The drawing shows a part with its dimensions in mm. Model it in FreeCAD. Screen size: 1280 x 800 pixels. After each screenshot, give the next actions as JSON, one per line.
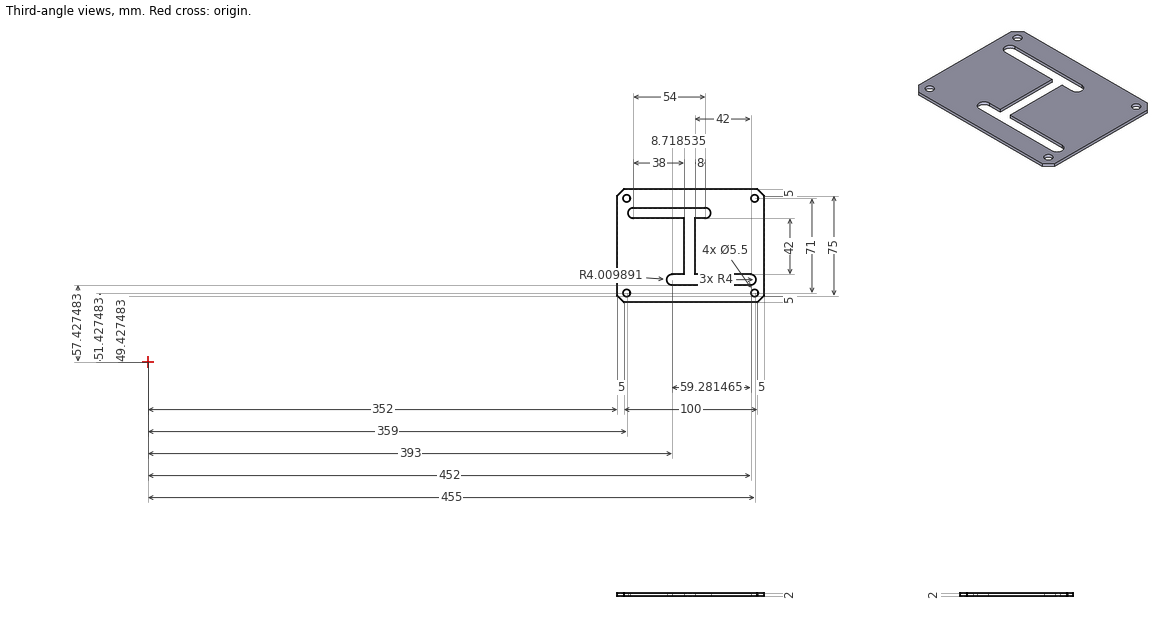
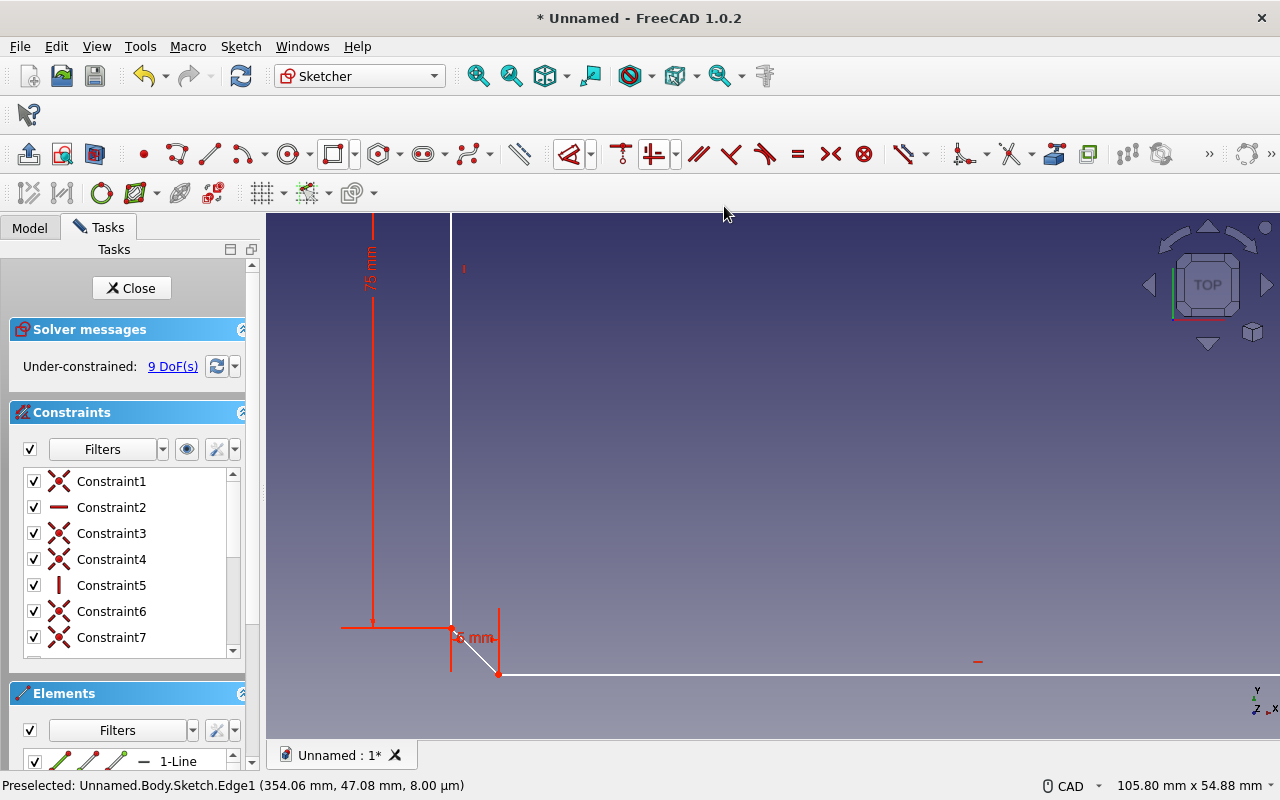
{"action": "left_click", "coordinate": [485, 661]}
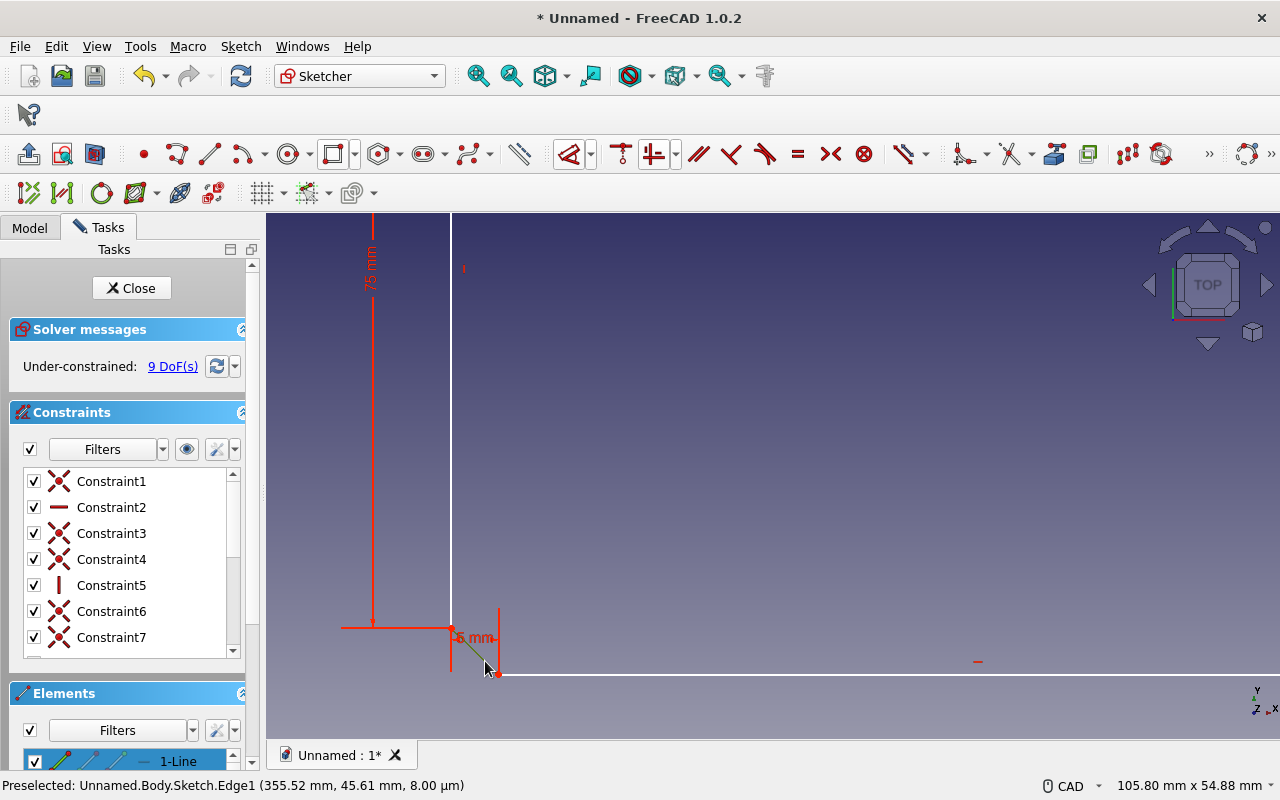
{"action": "key", "text": "i"}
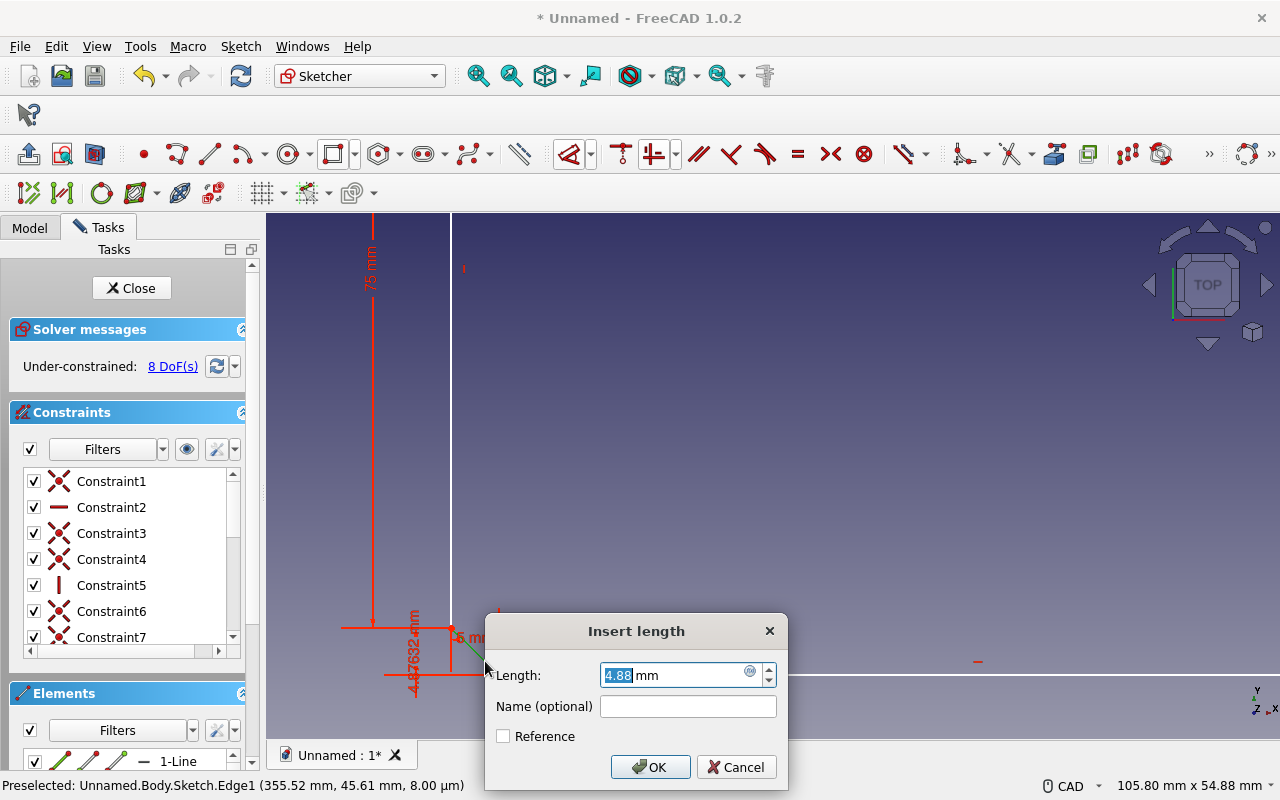
{"action": "type", "text": "5"}
{"action": "key", "text": "Return"}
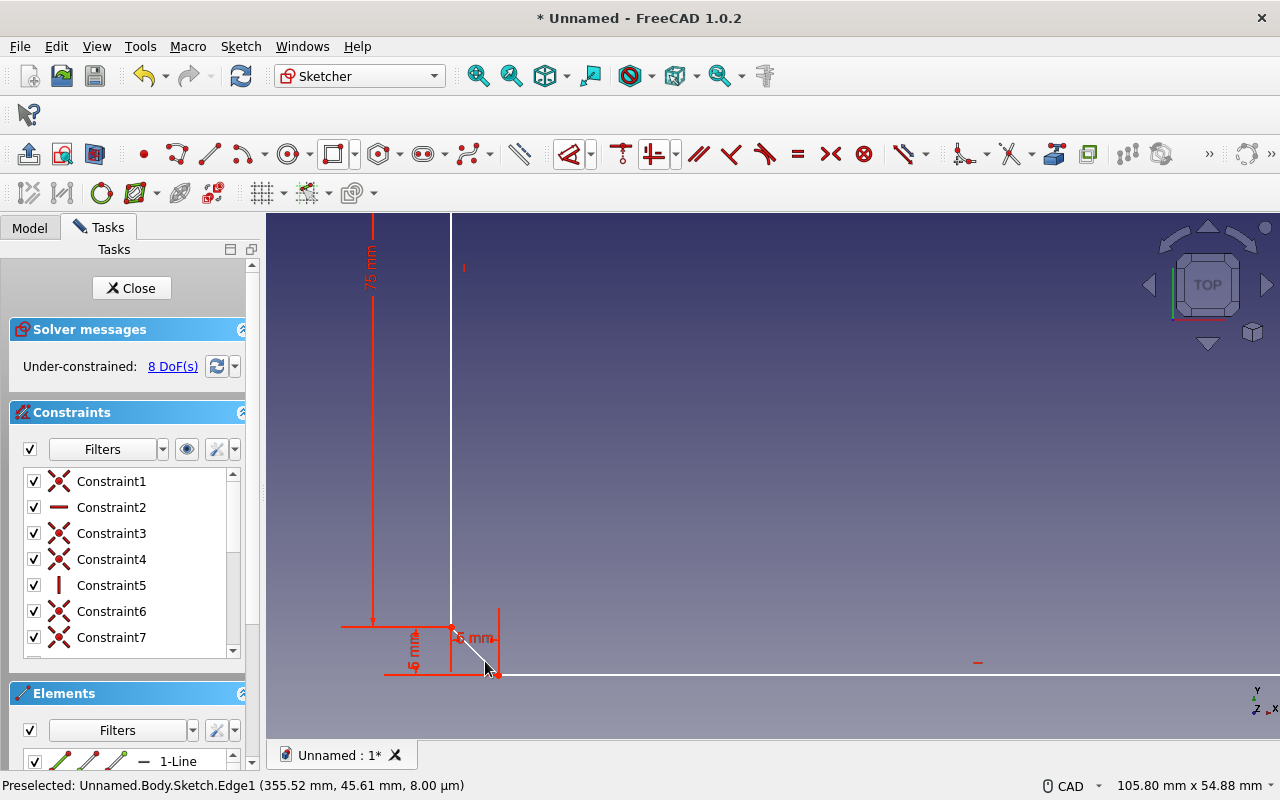
{"action": "scroll", "coordinate": [481, 648], "scroll_direction": "down", "scroll_amount": 4}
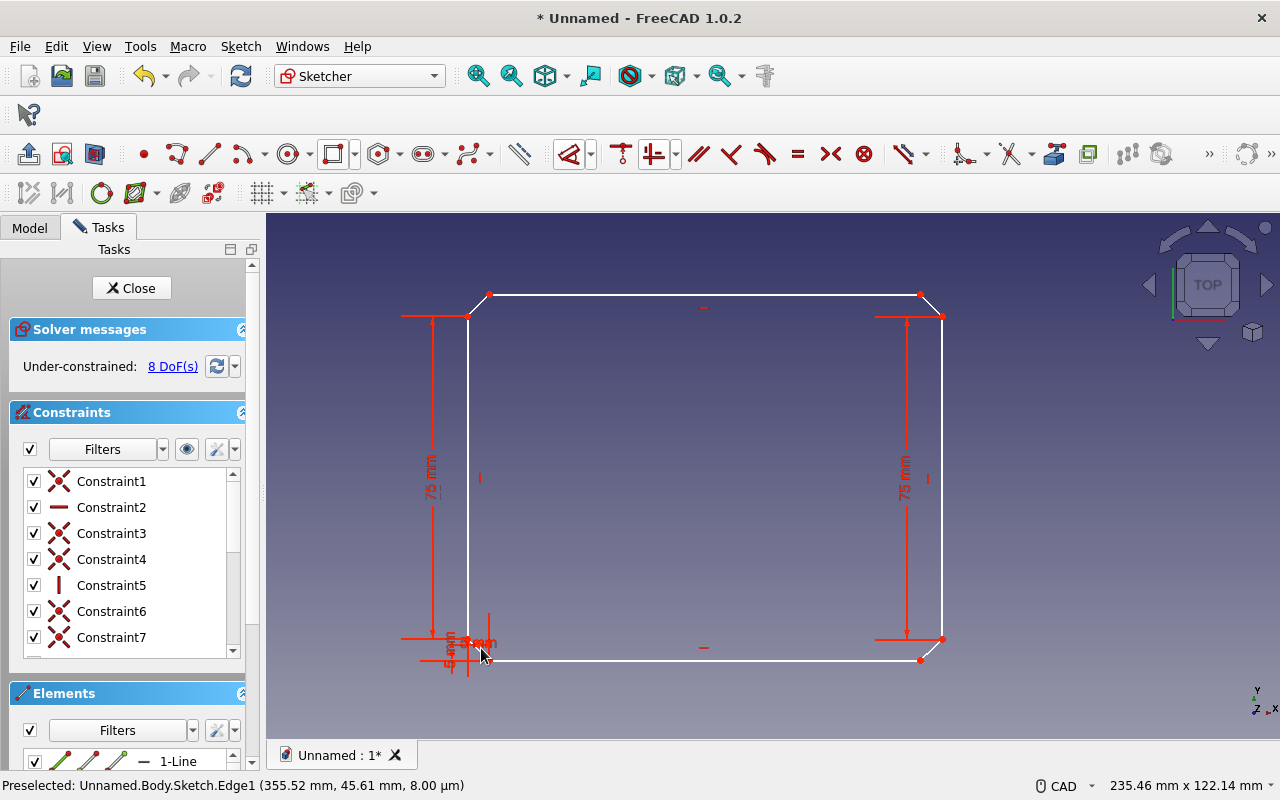
{"action": "scroll", "coordinate": [927, 654], "scroll_direction": "up", "scroll_amount": 4}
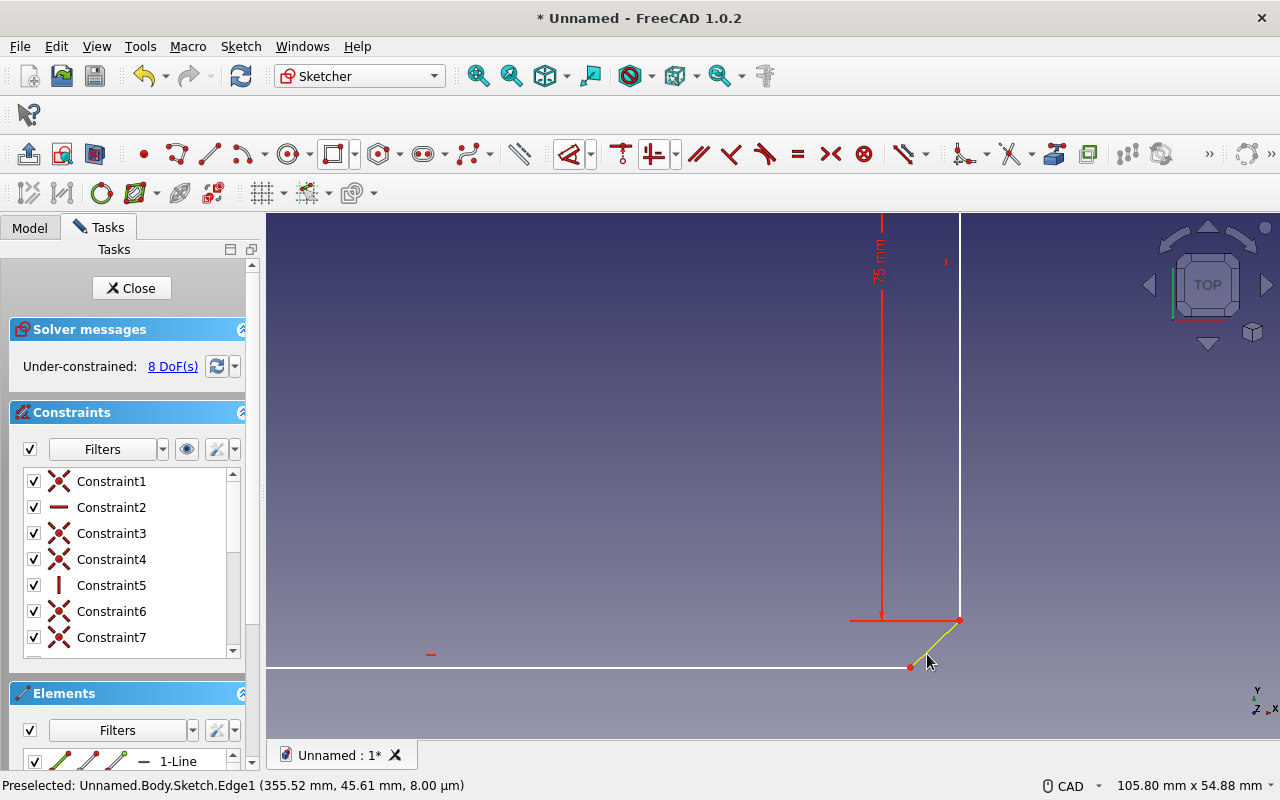
{"action": "left_click", "coordinate": [925, 654]}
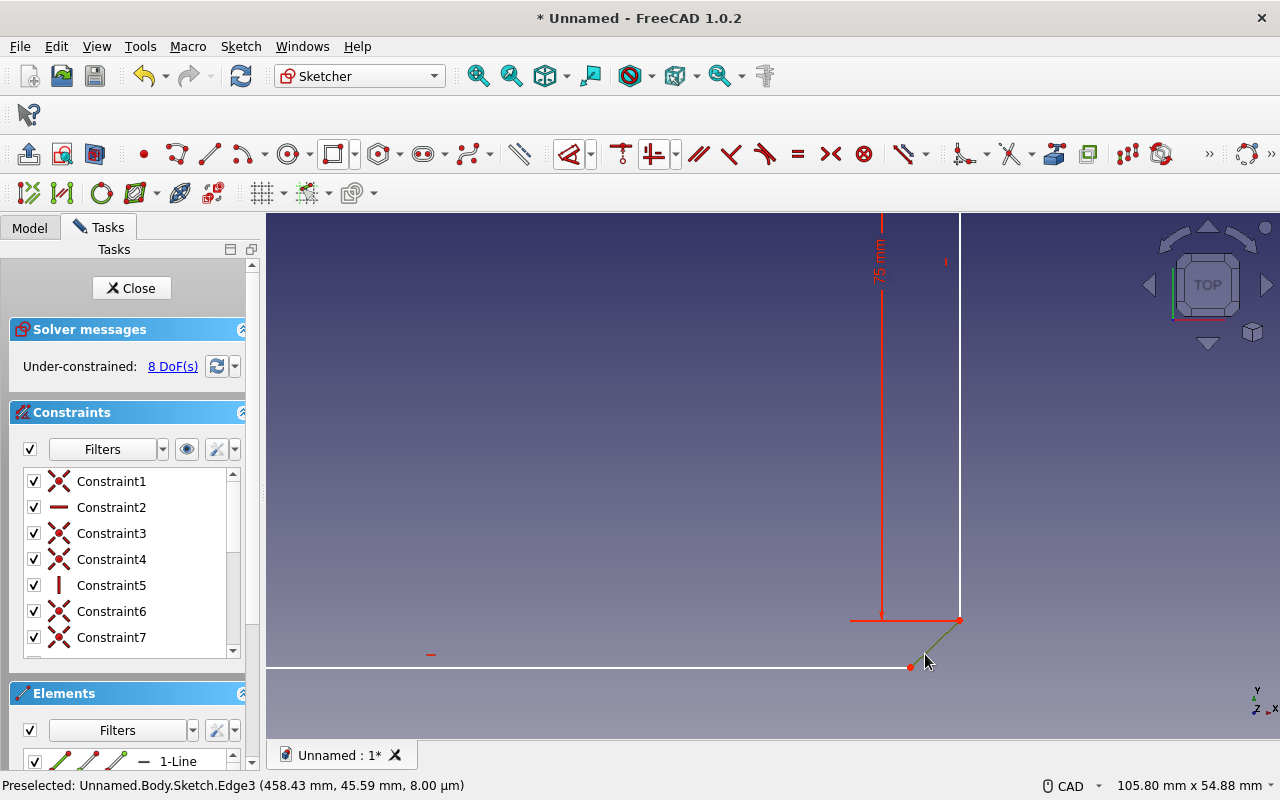
{"action": "key", "text": "l"}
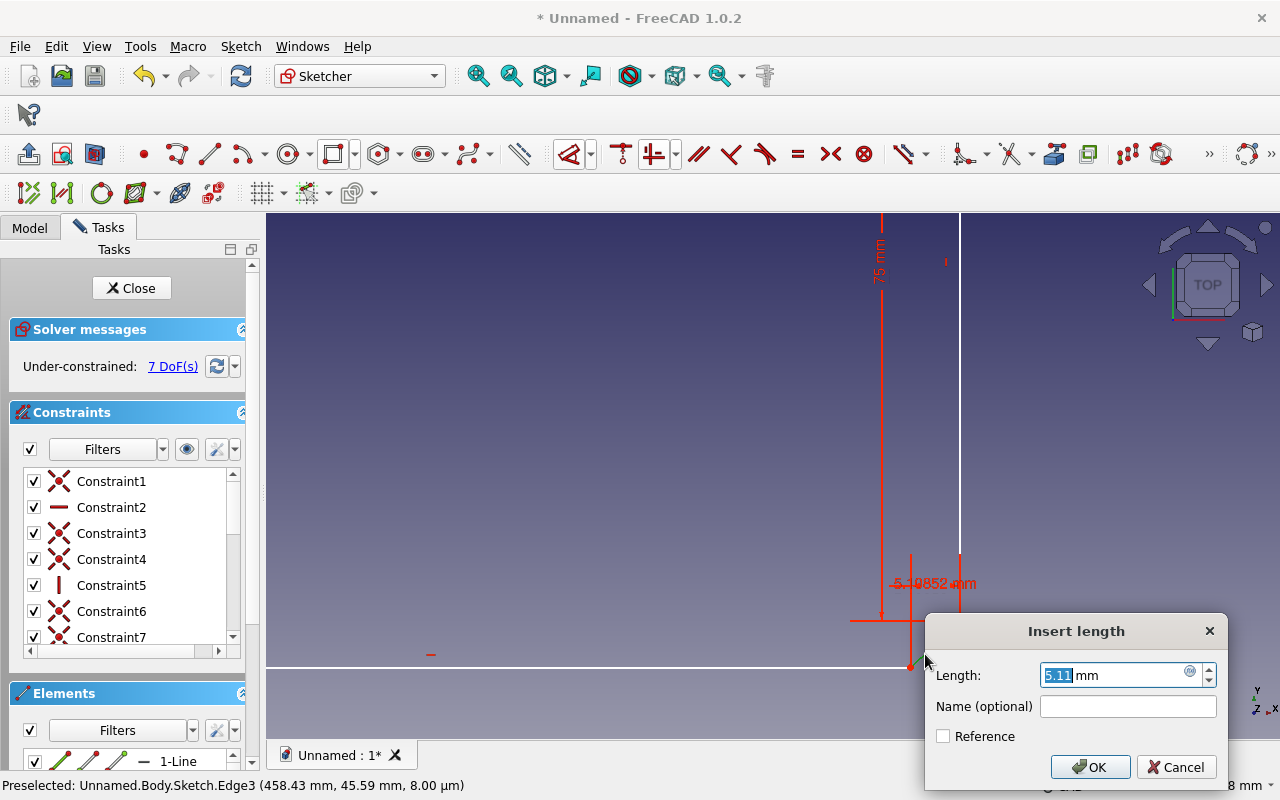
{"action": "type", "text": "5"}
{"action": "key", "text": "Return"}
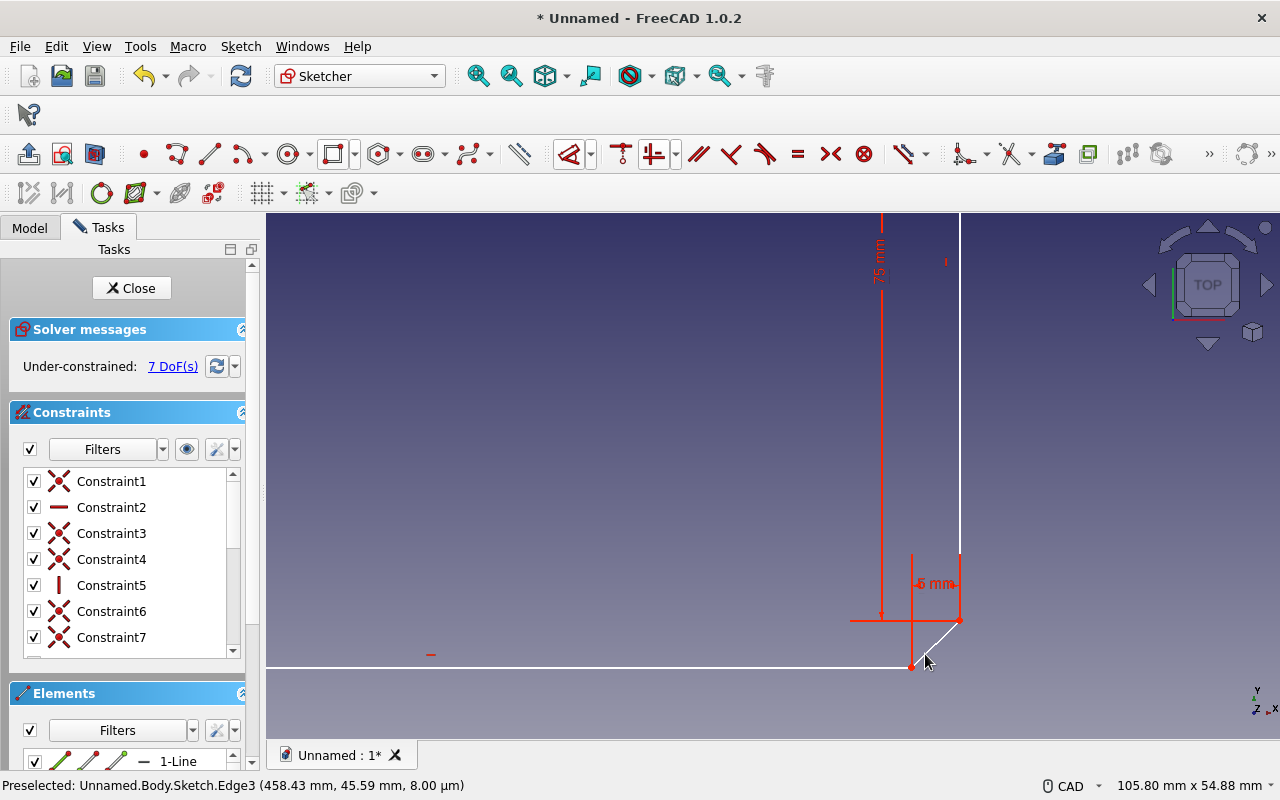
{"action": "left_click", "coordinate": [926, 654]}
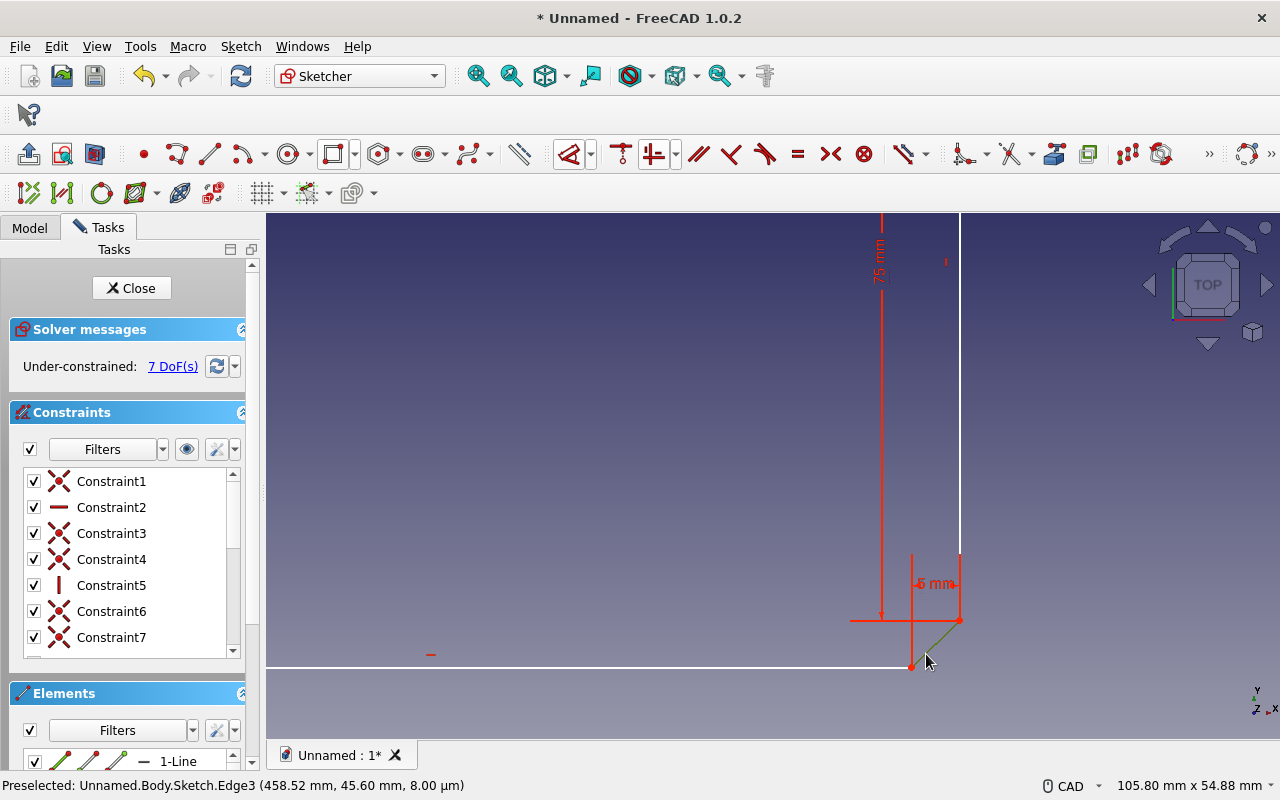
{"action": "key", "text": "i"}